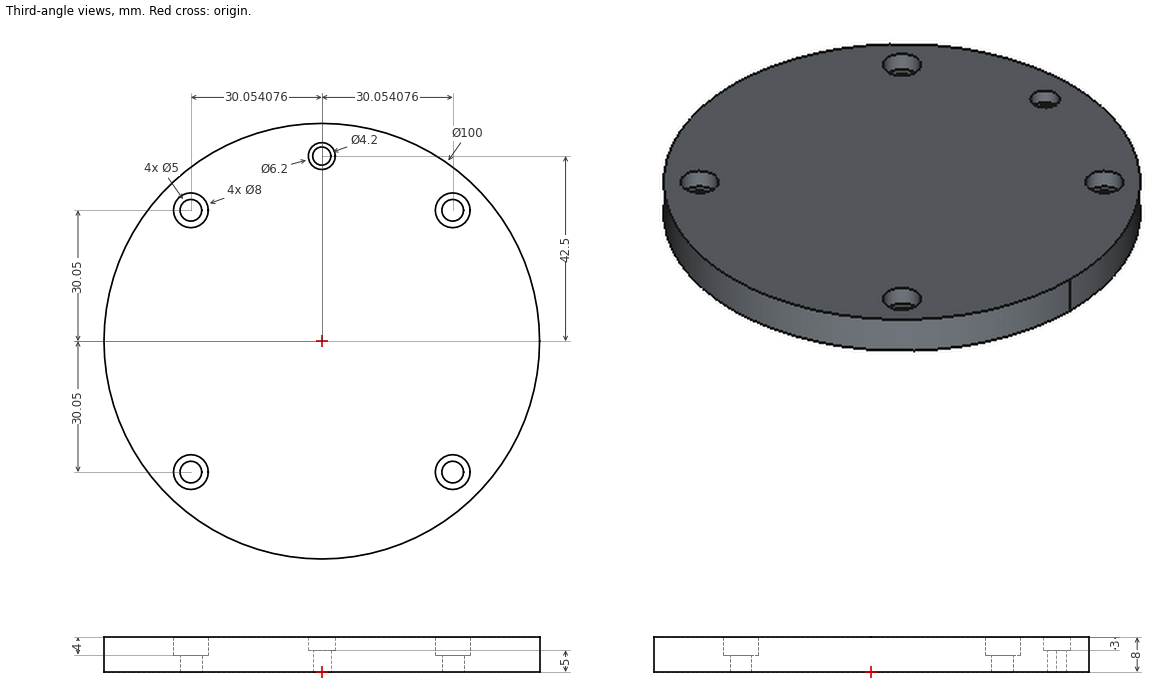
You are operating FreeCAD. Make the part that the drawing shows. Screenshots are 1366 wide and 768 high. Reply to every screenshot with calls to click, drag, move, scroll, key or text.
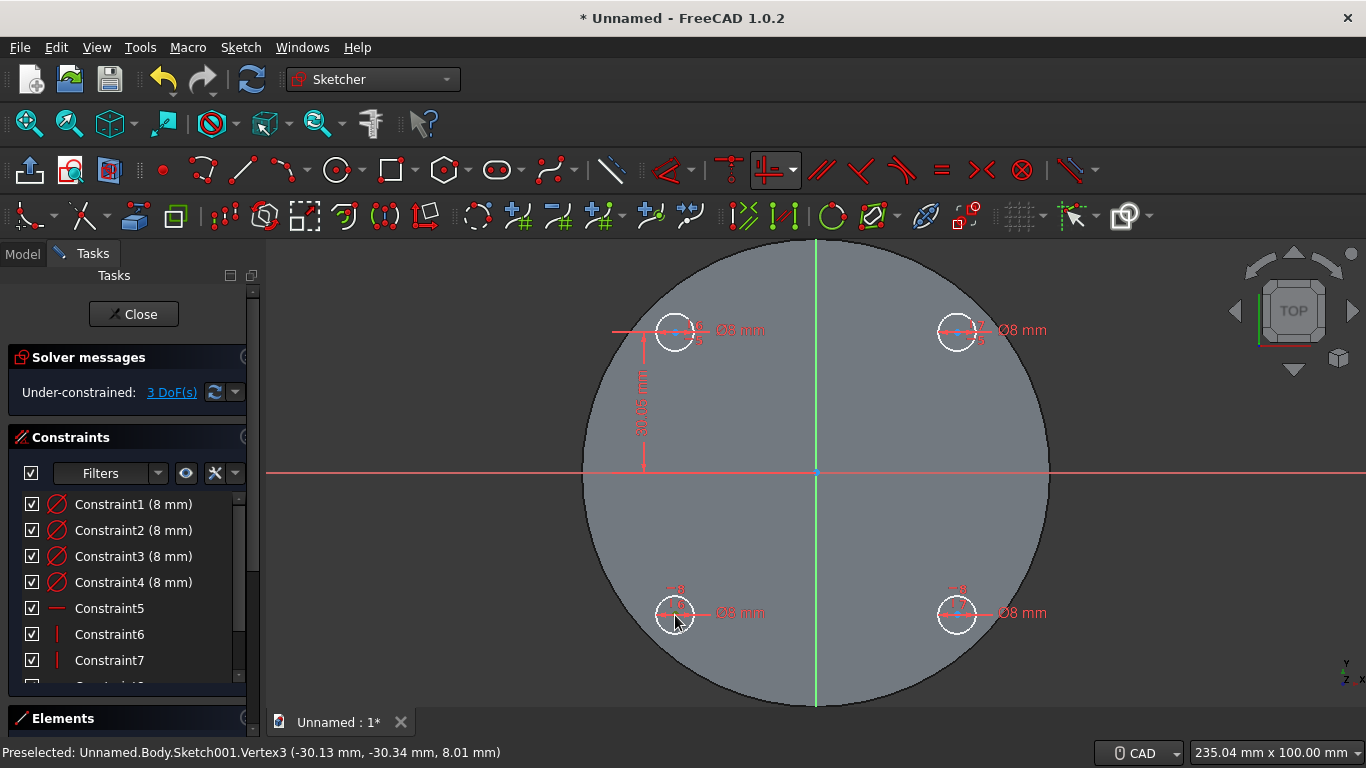
click(694, 170)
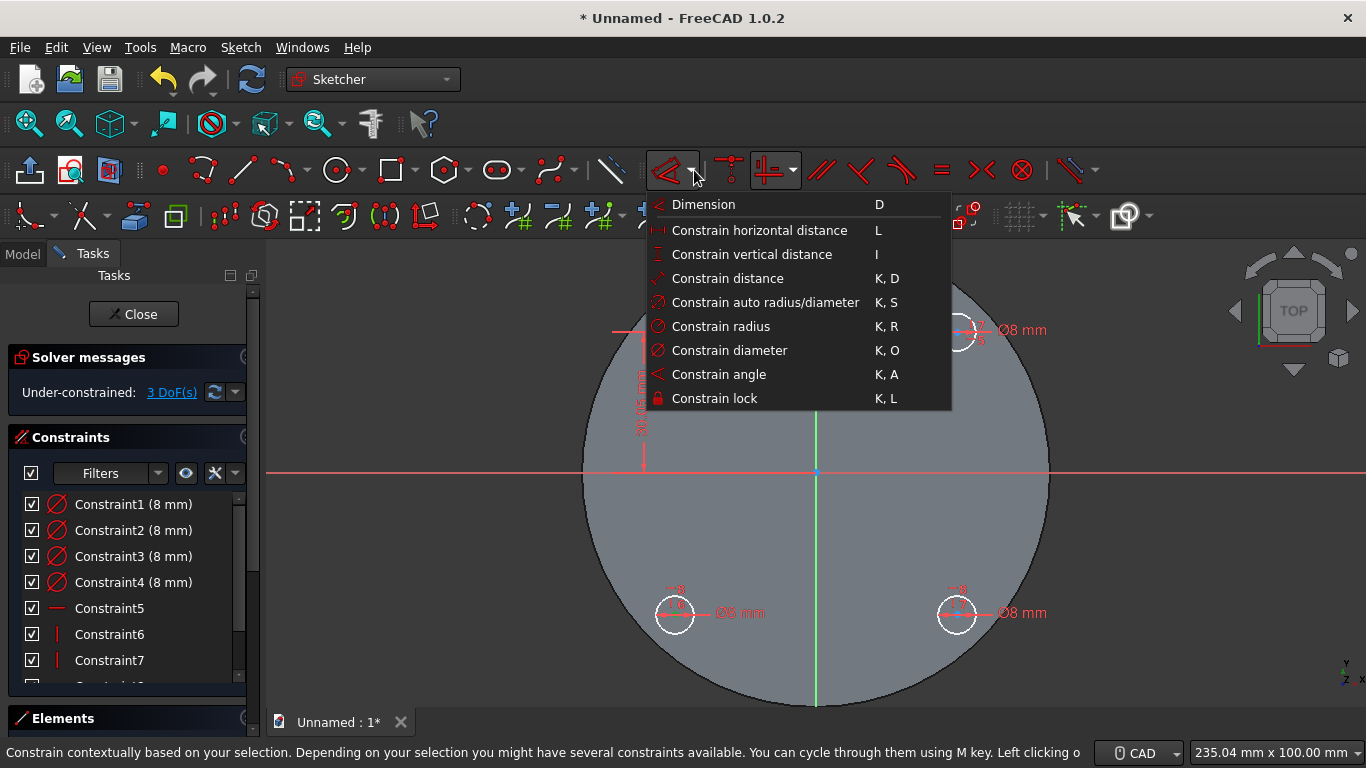
click(799, 254)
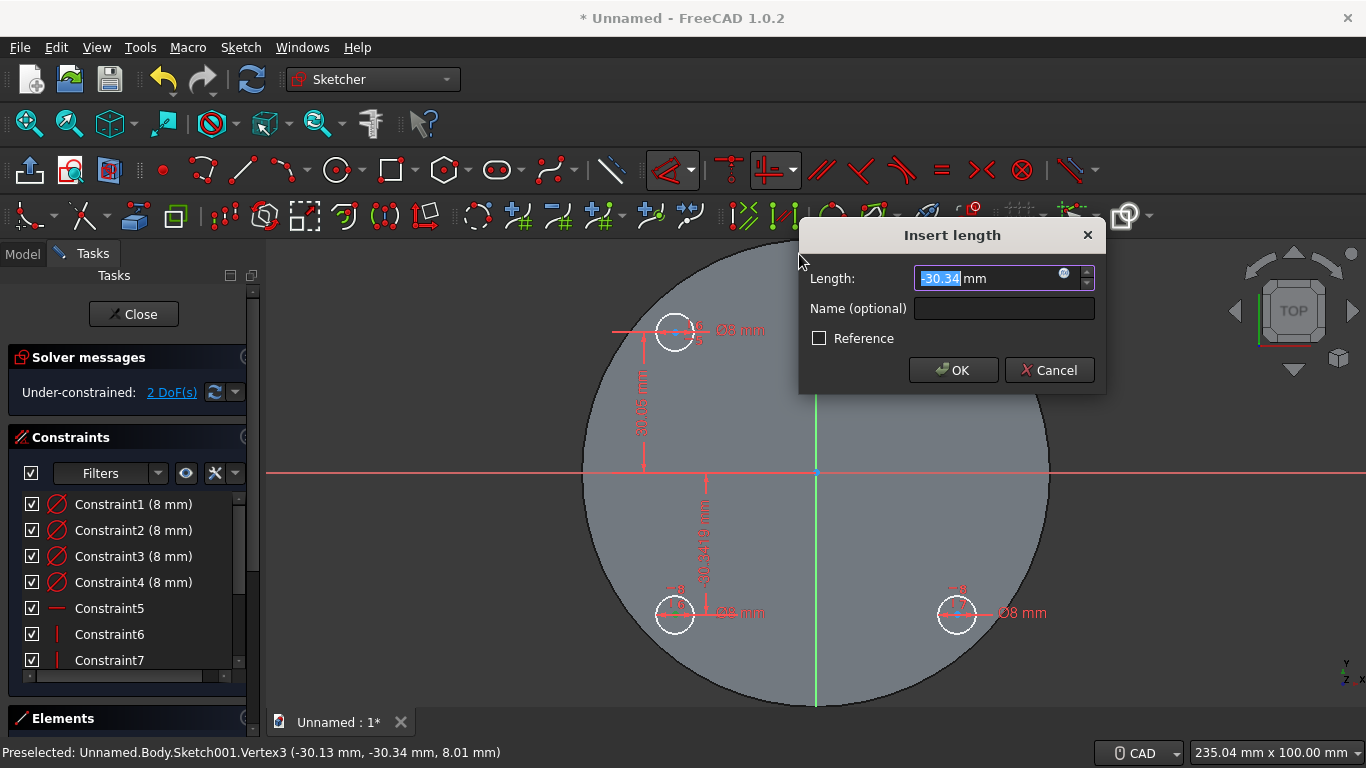
text(-30.05)
key(Return)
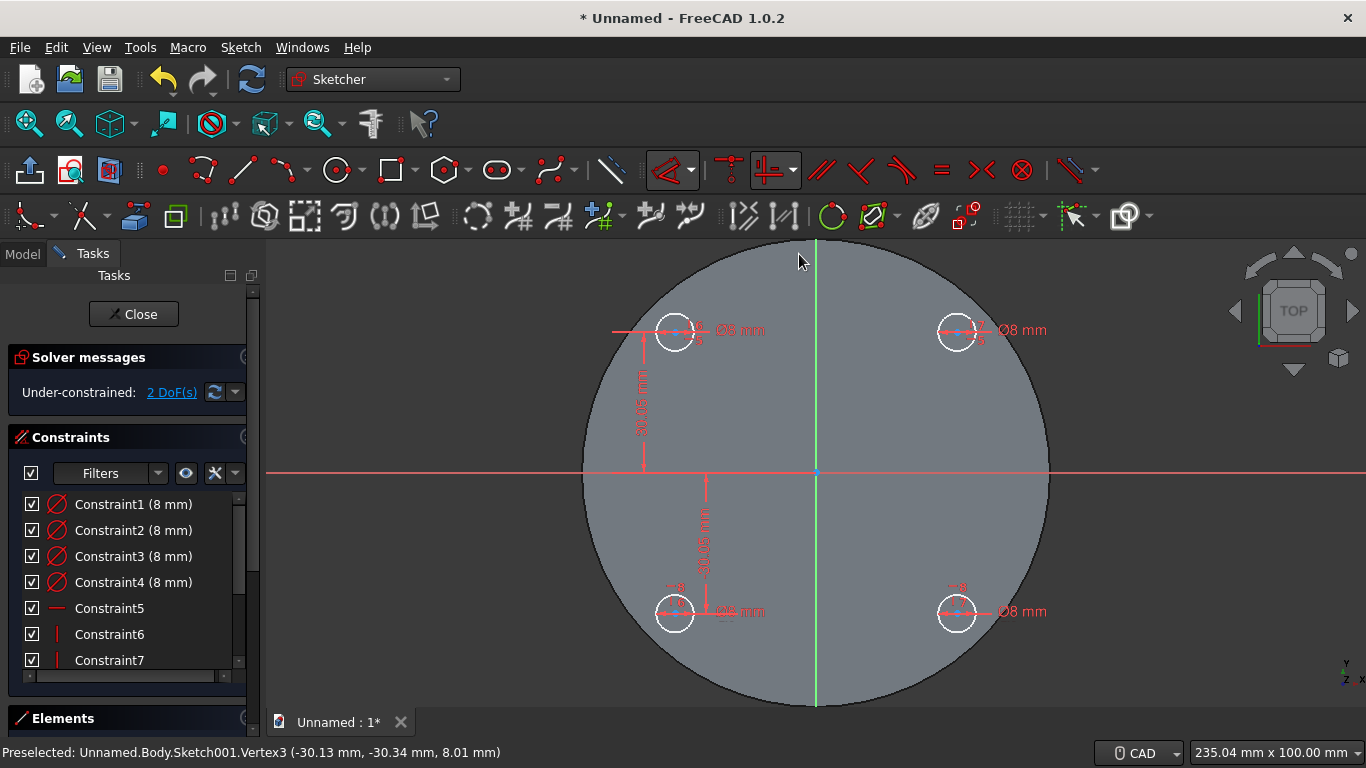
click(675, 332)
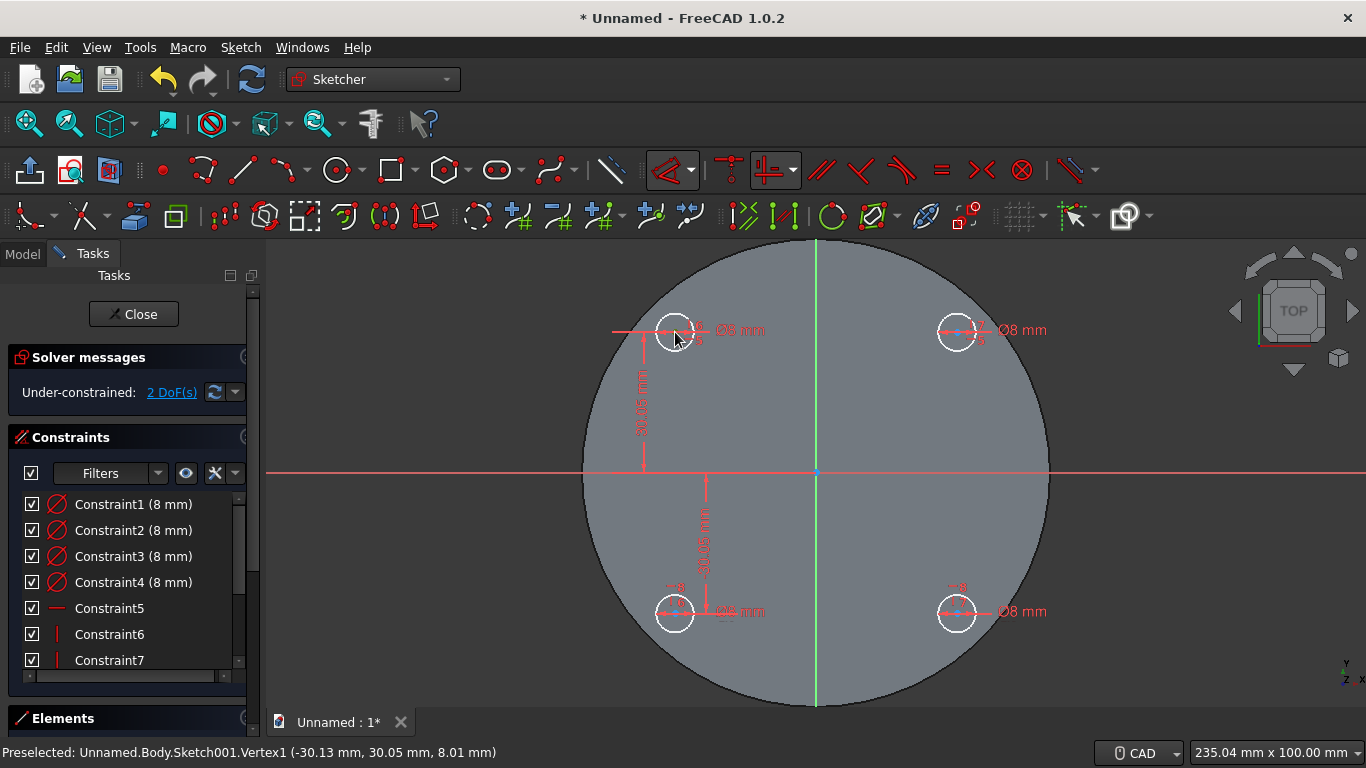
key(l)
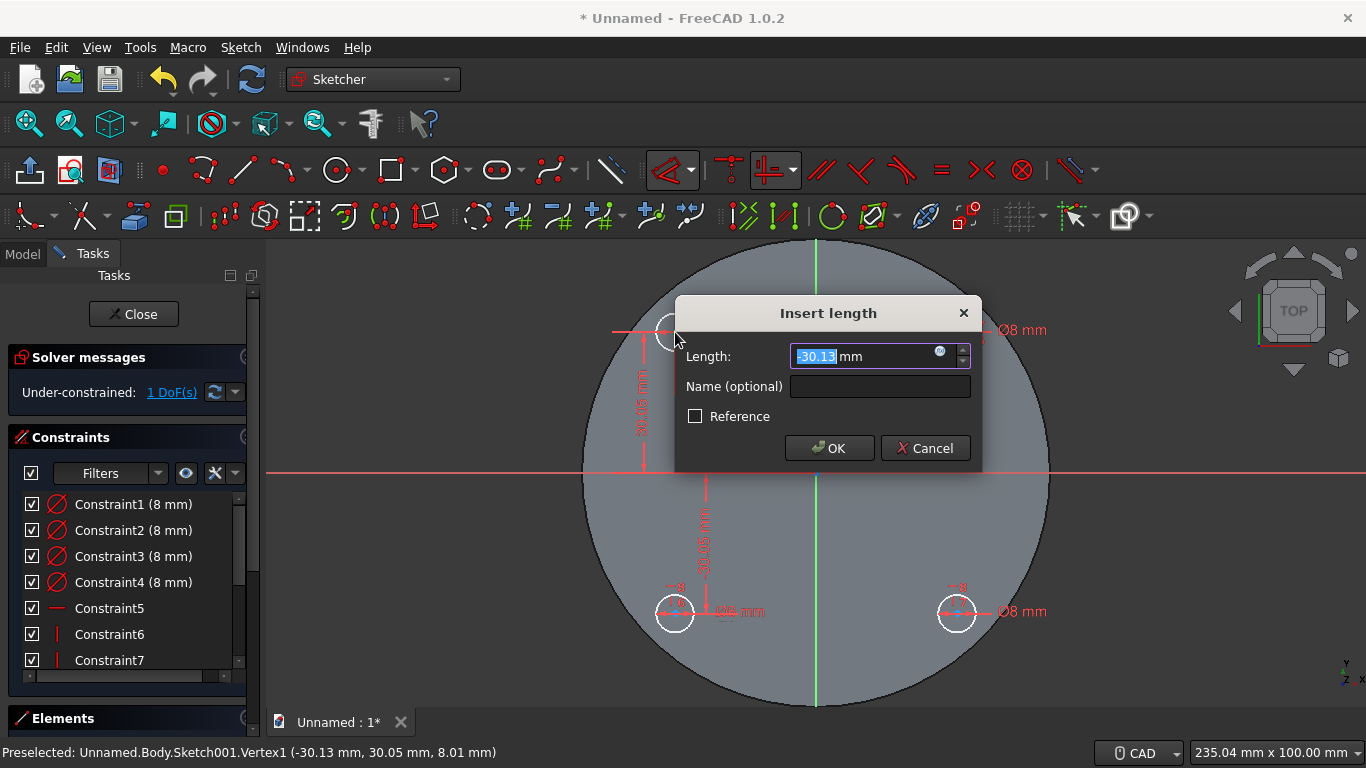
text(-30.054076)
key(Return)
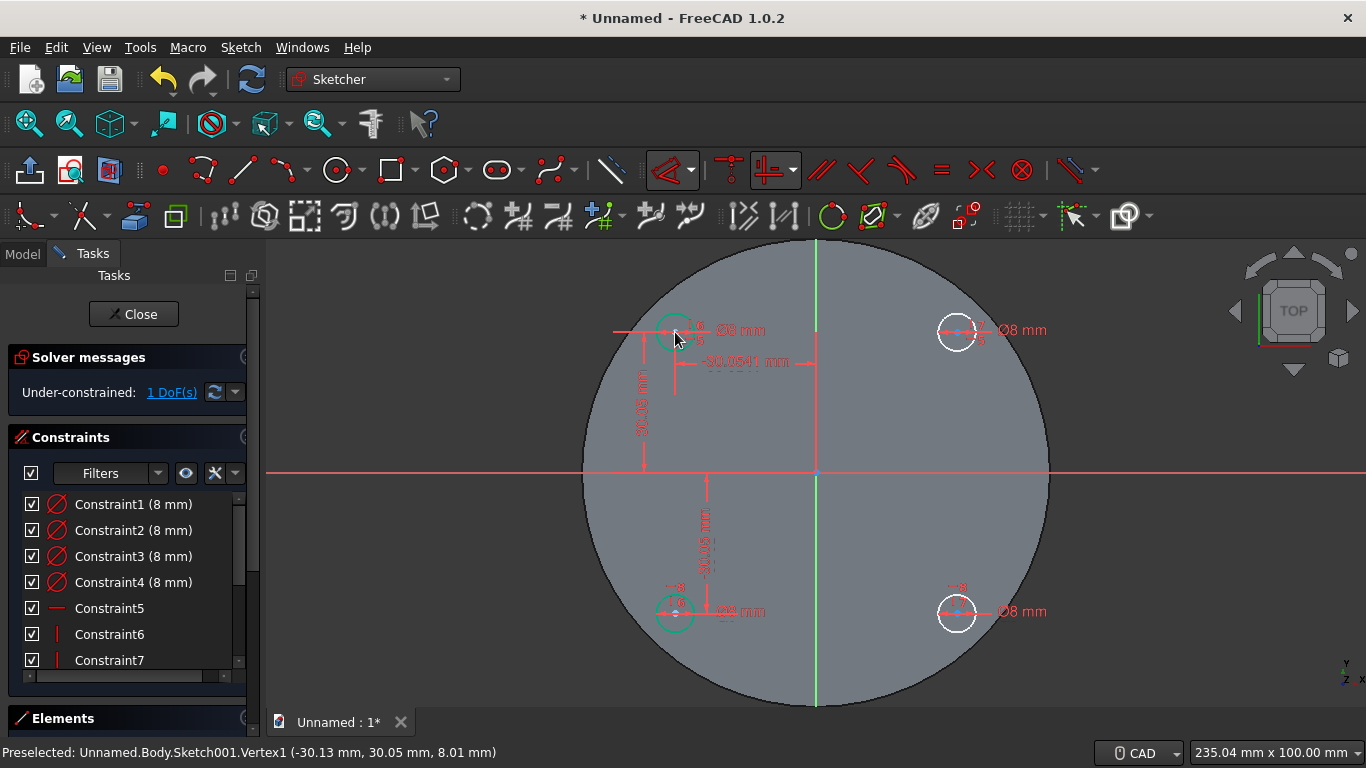
click(957, 332)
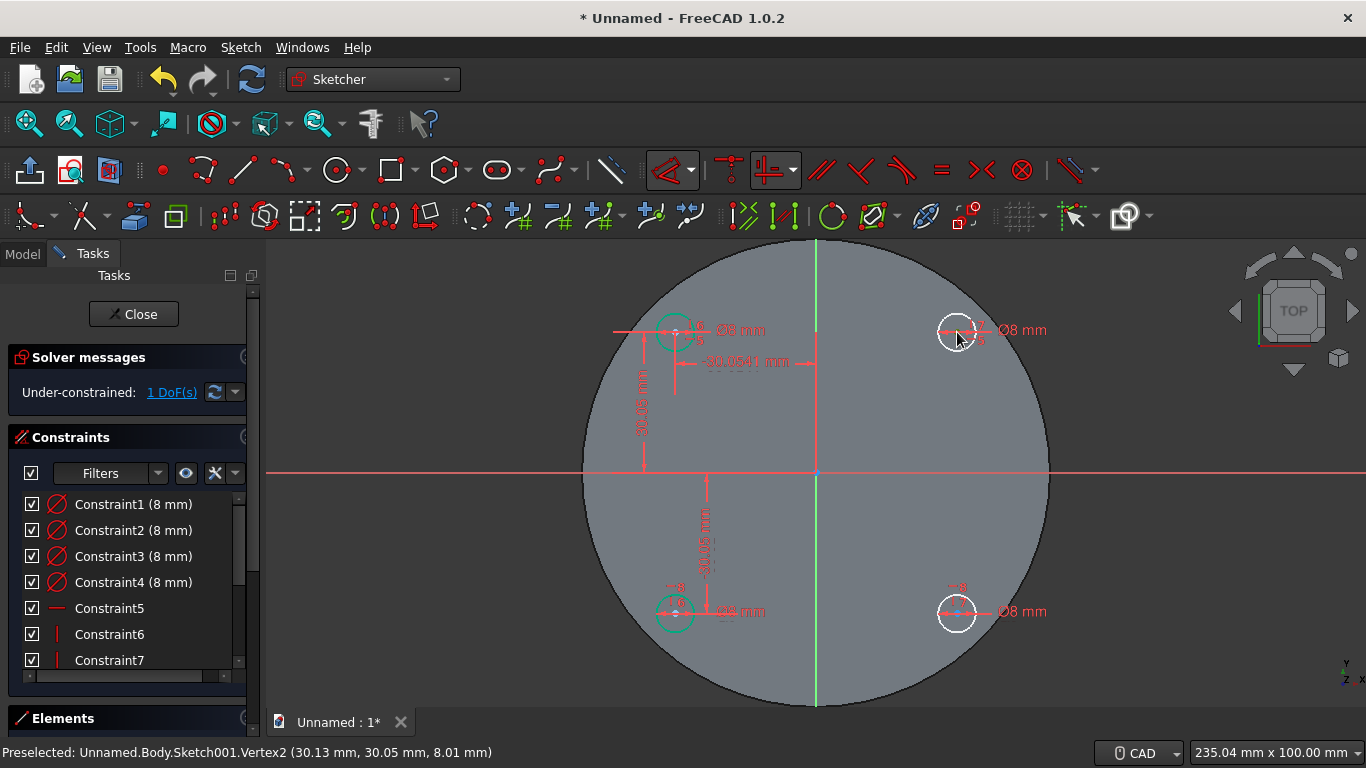
key(l)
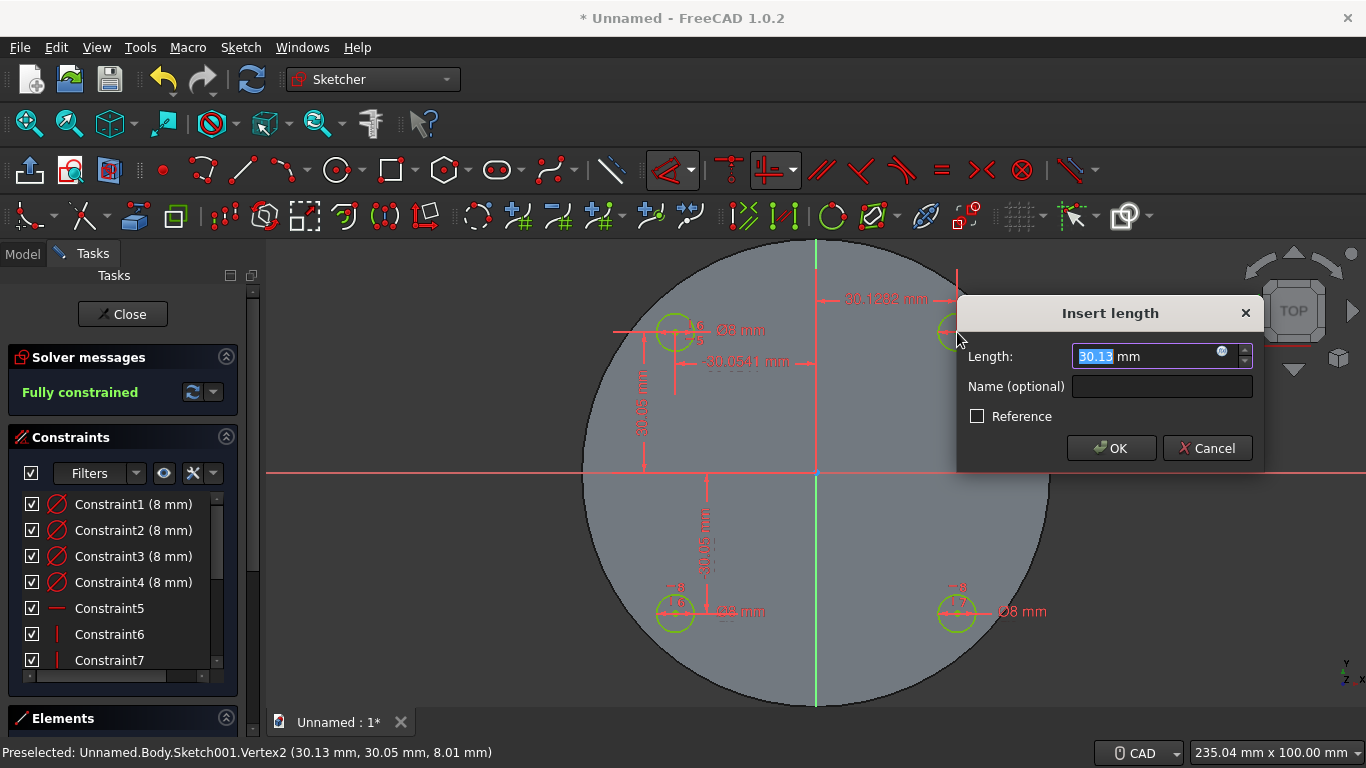
text(30.054076)
key(Return)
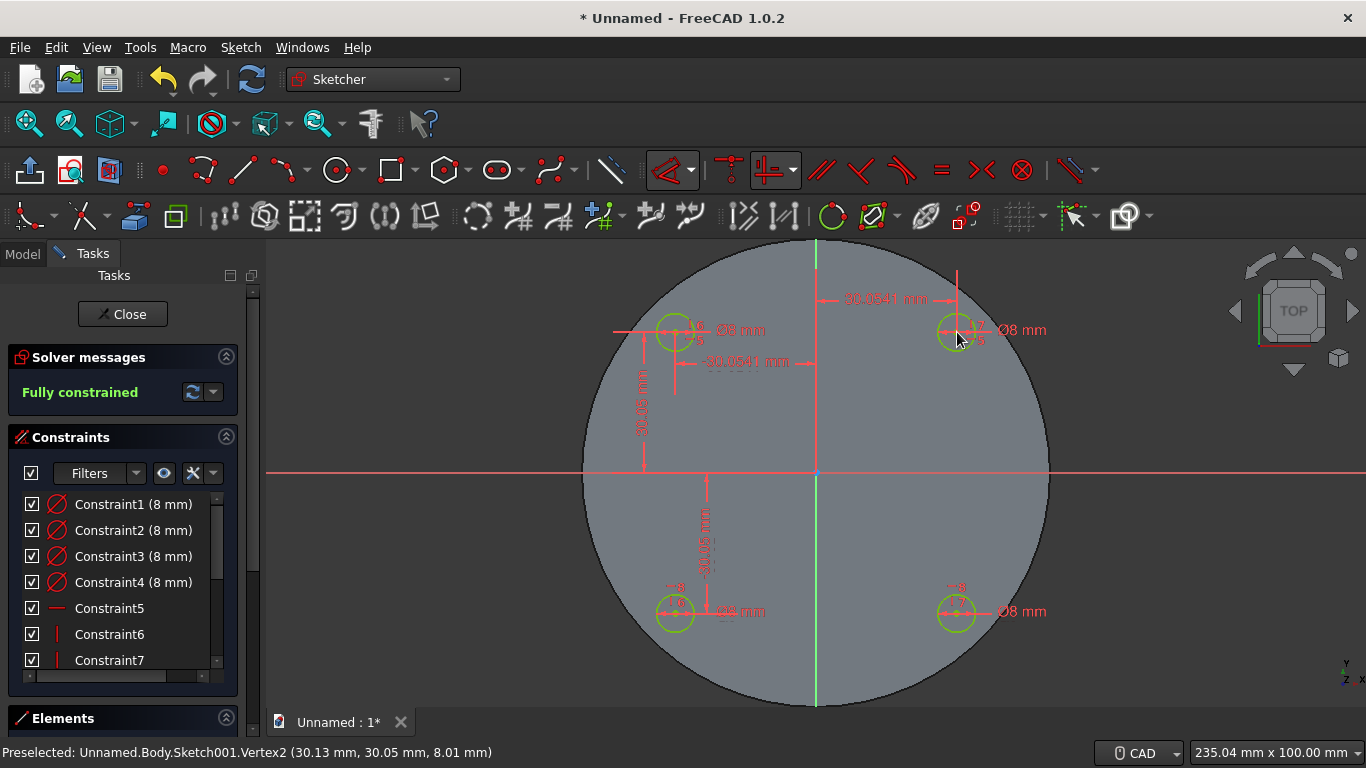
click(123, 314)